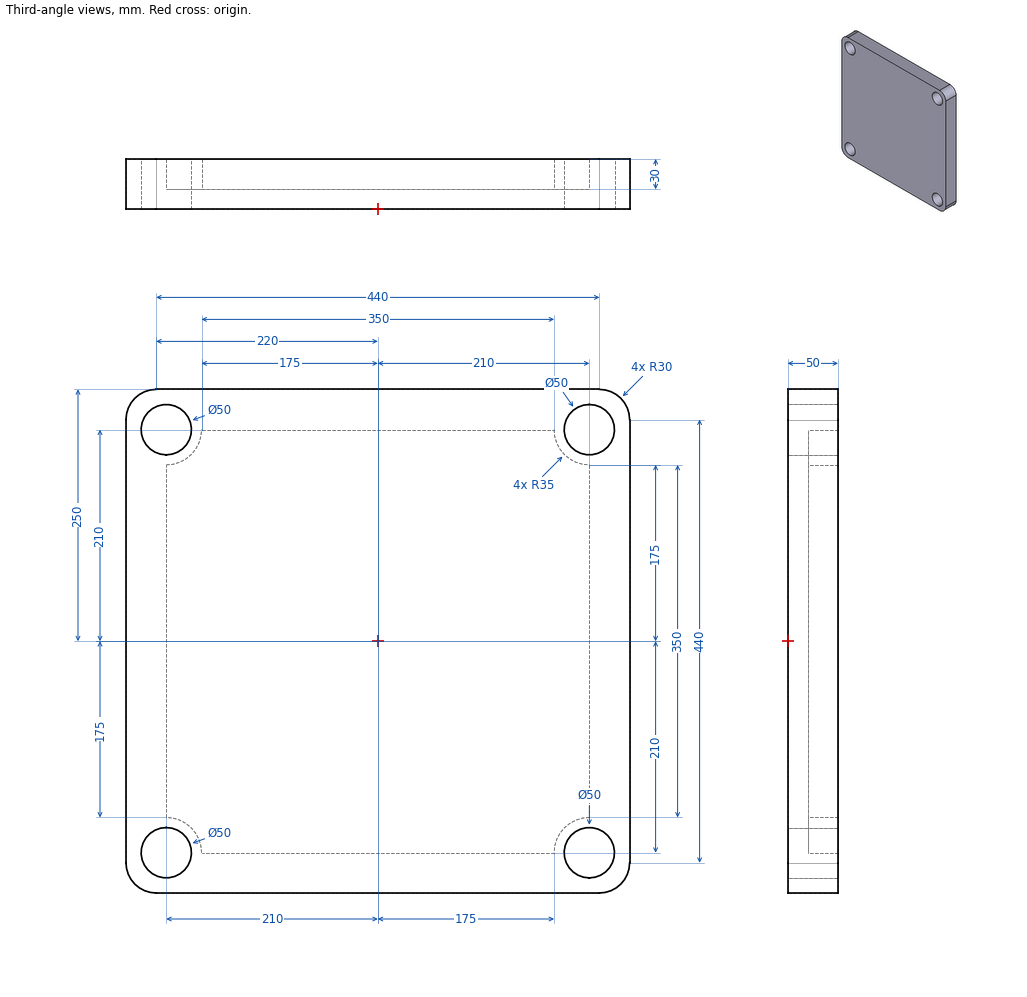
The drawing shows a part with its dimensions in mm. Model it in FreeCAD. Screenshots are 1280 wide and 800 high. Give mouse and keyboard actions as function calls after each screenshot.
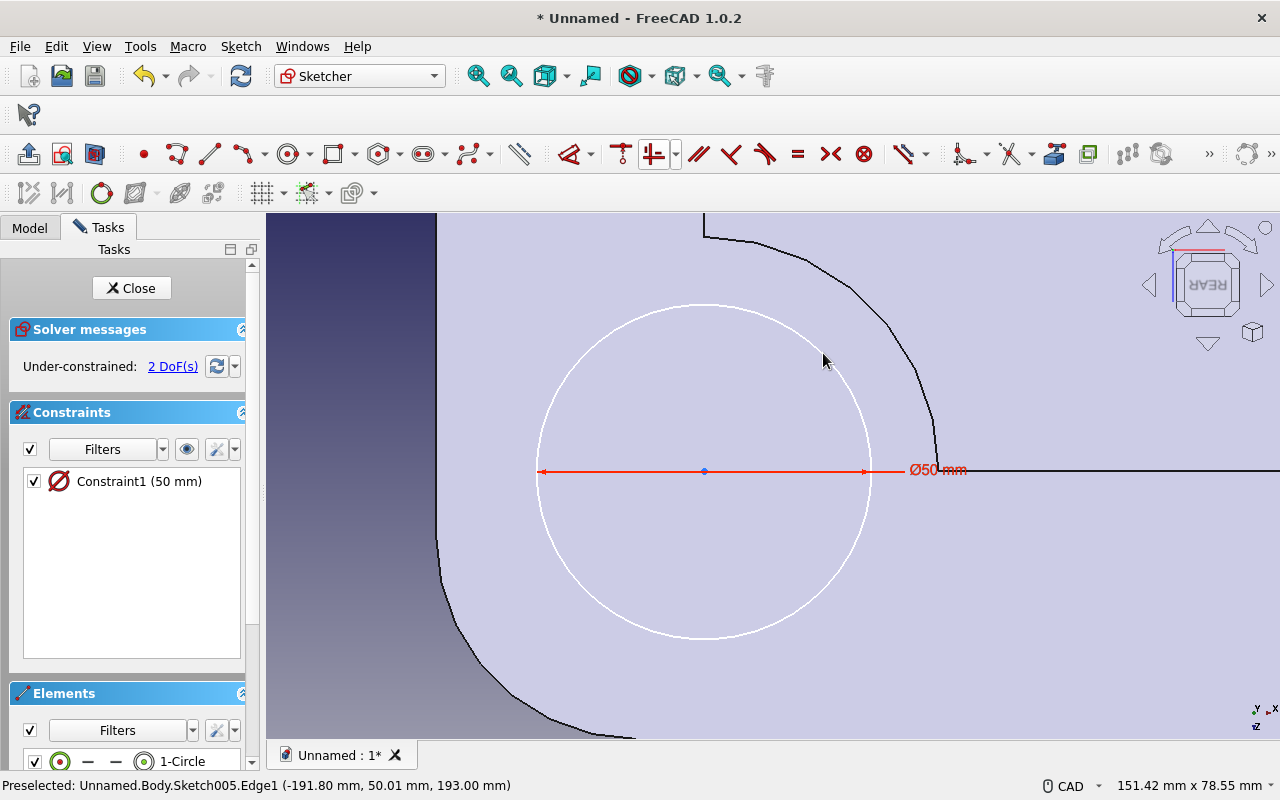
click(568, 154)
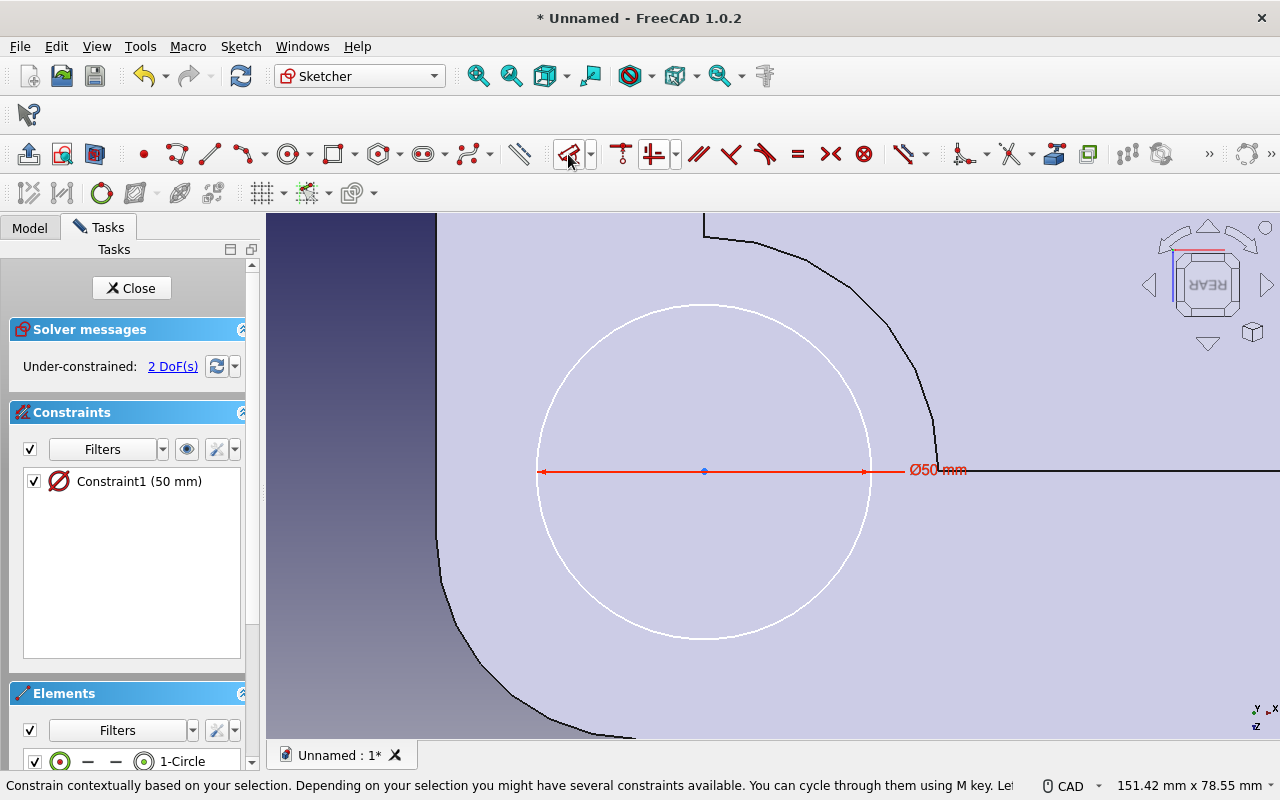
click(704, 472)
click(909, 506)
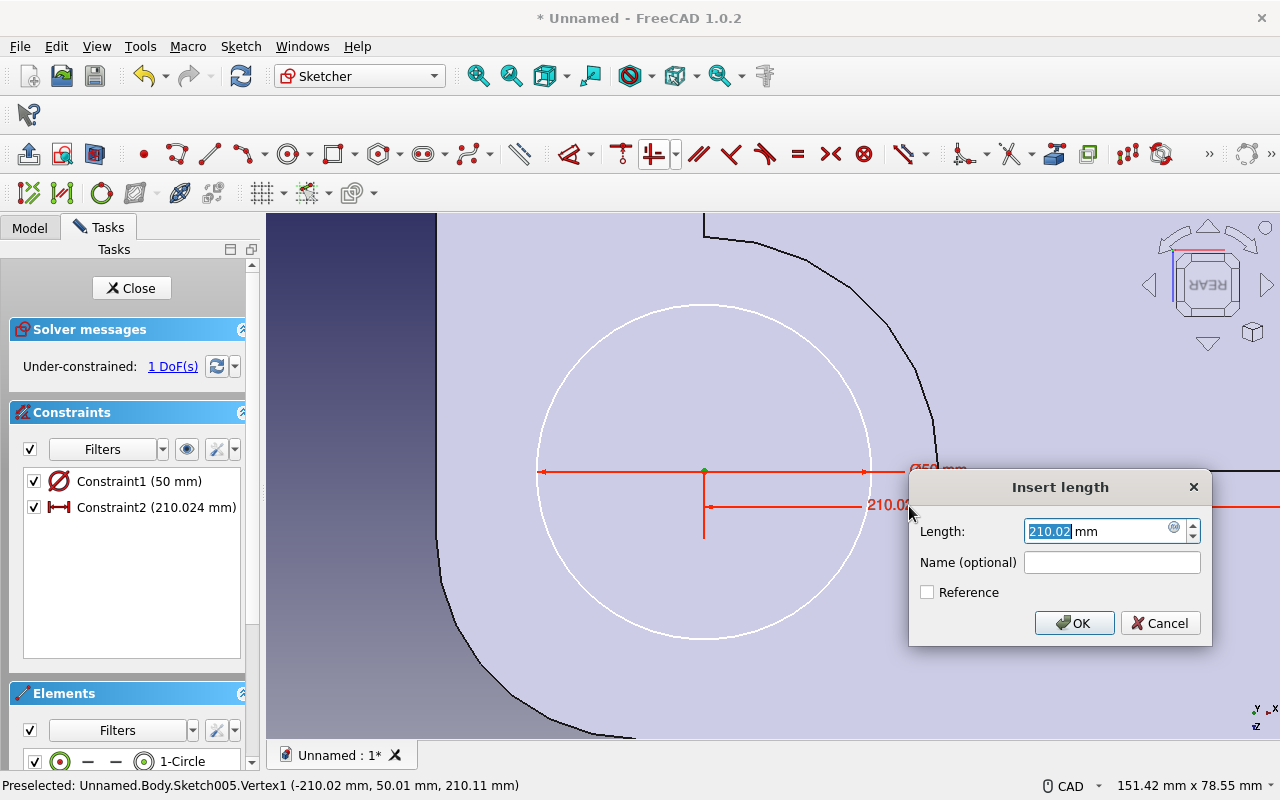
text(210)
key(Return)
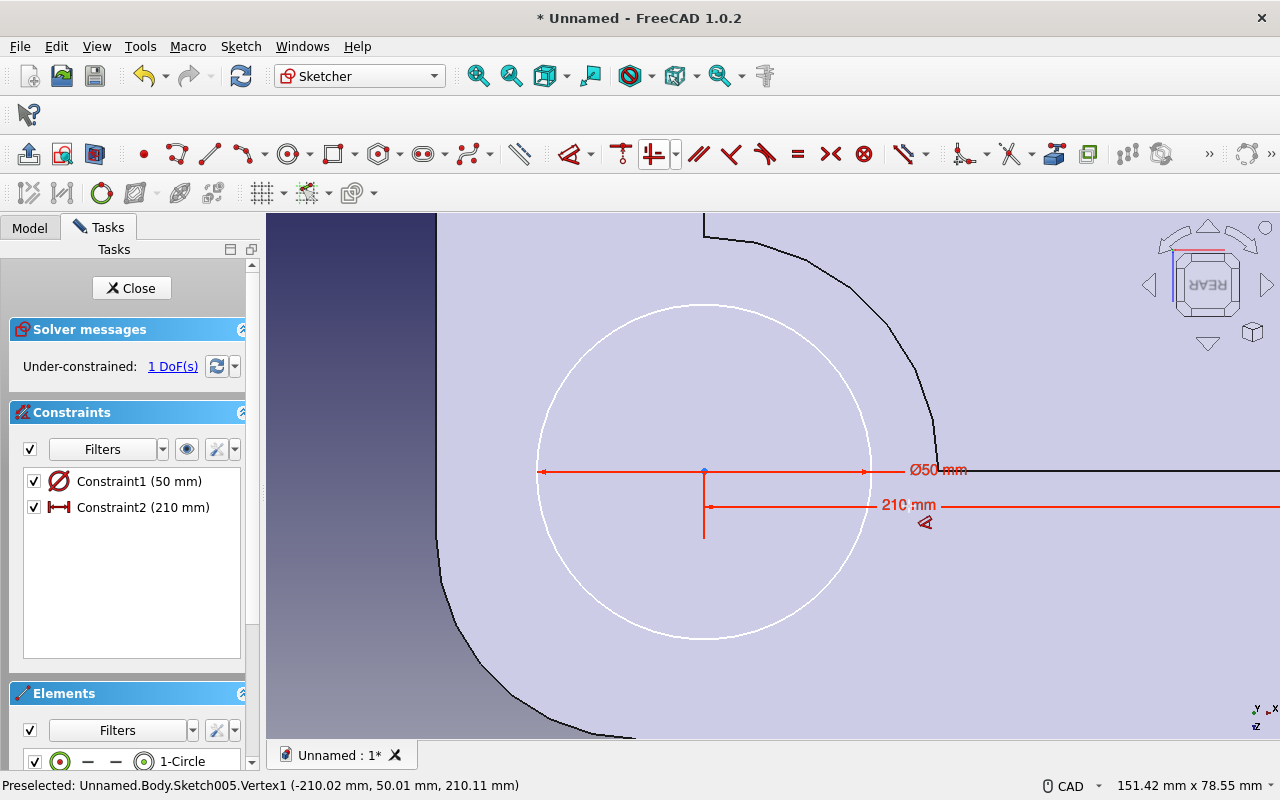
click(704, 472)
click(670, 356)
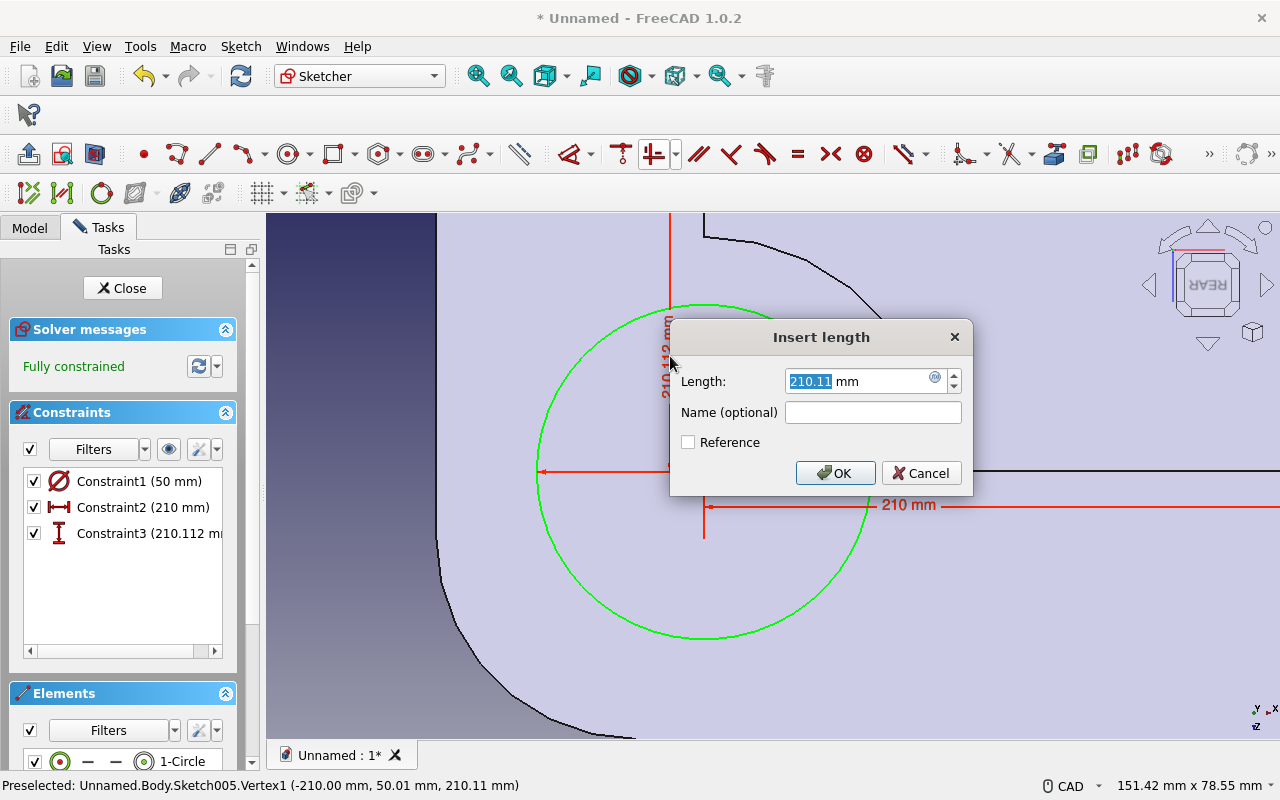
text(210)
key(Return)
key(Escape)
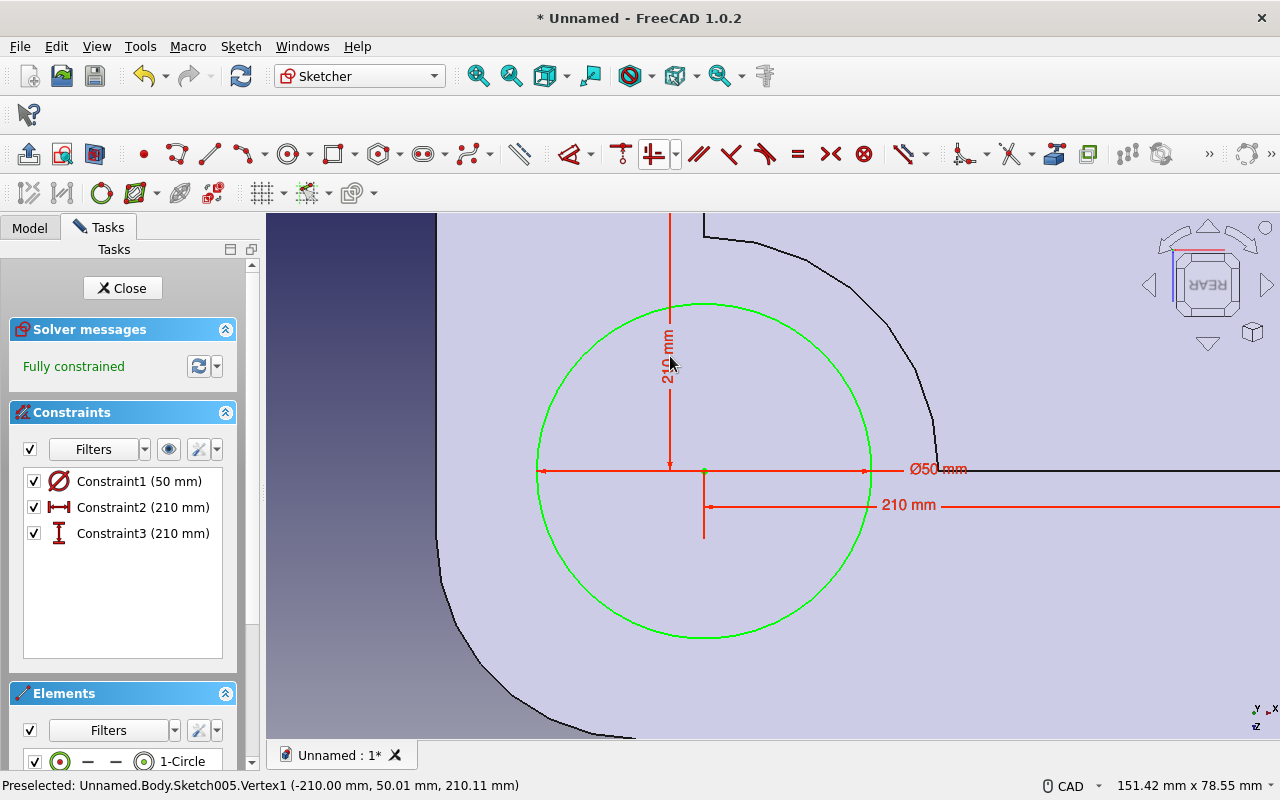
click(123, 288)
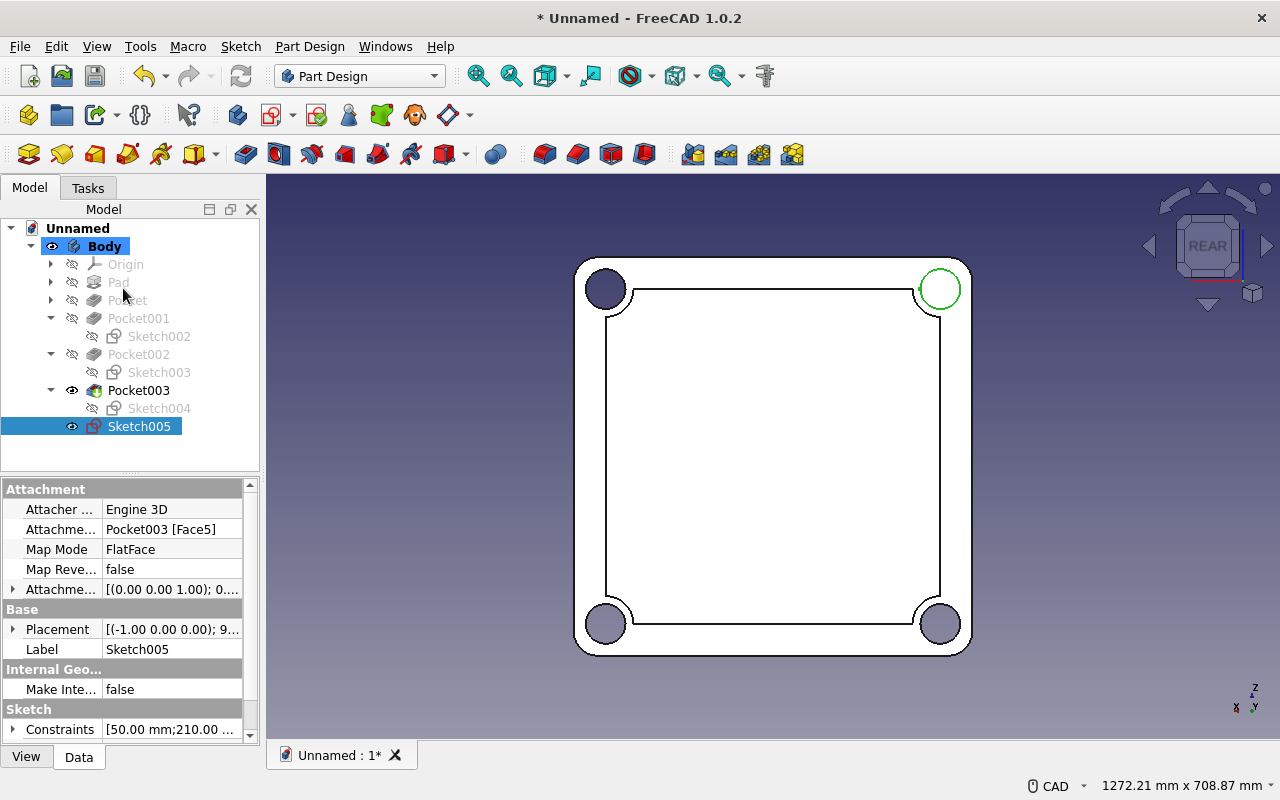
click(246, 154)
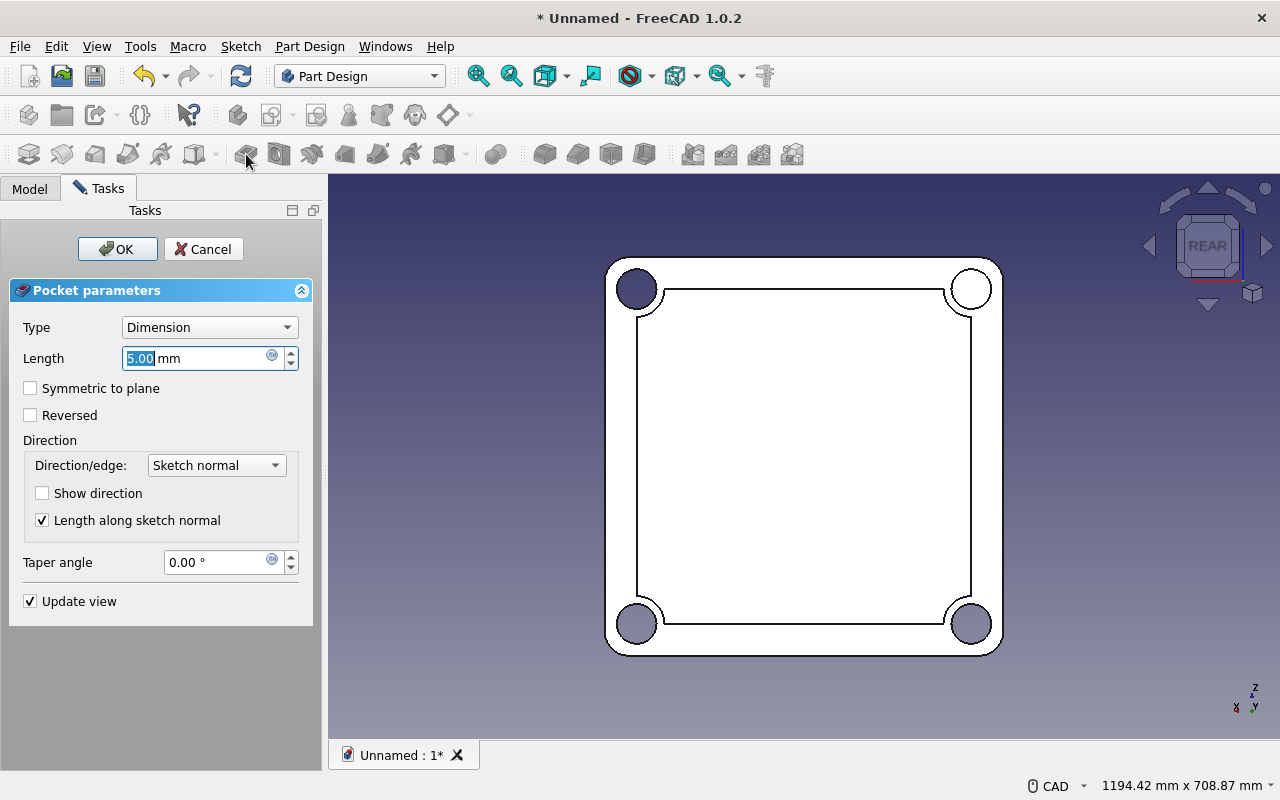
click(210, 328)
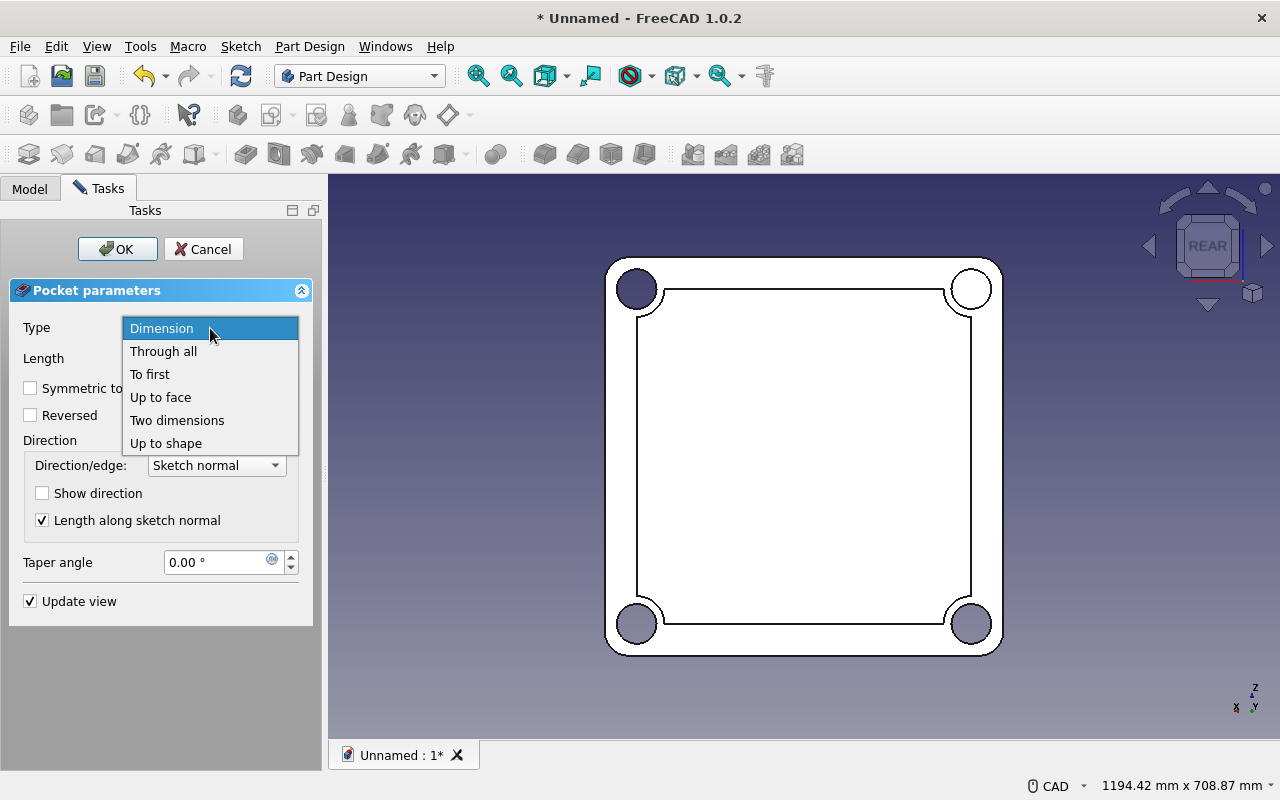
click(208, 374)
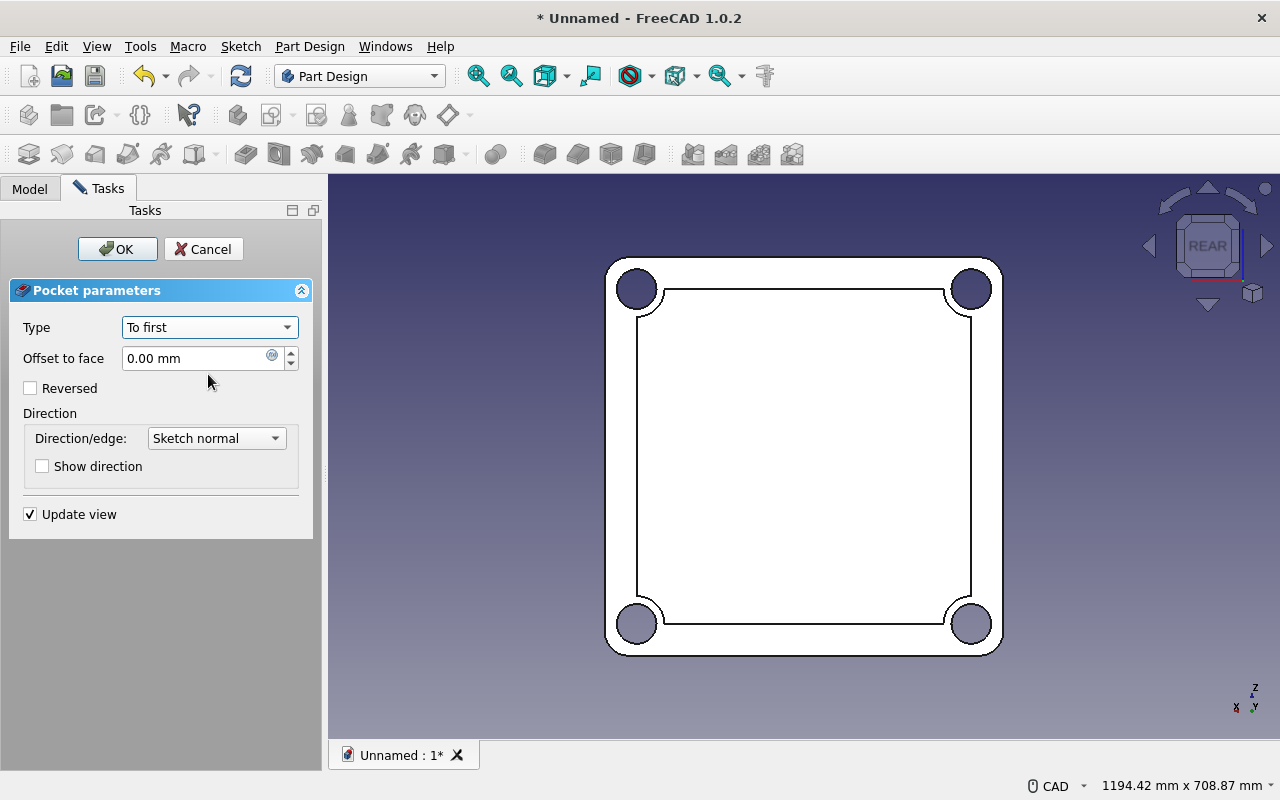
click(118, 249)